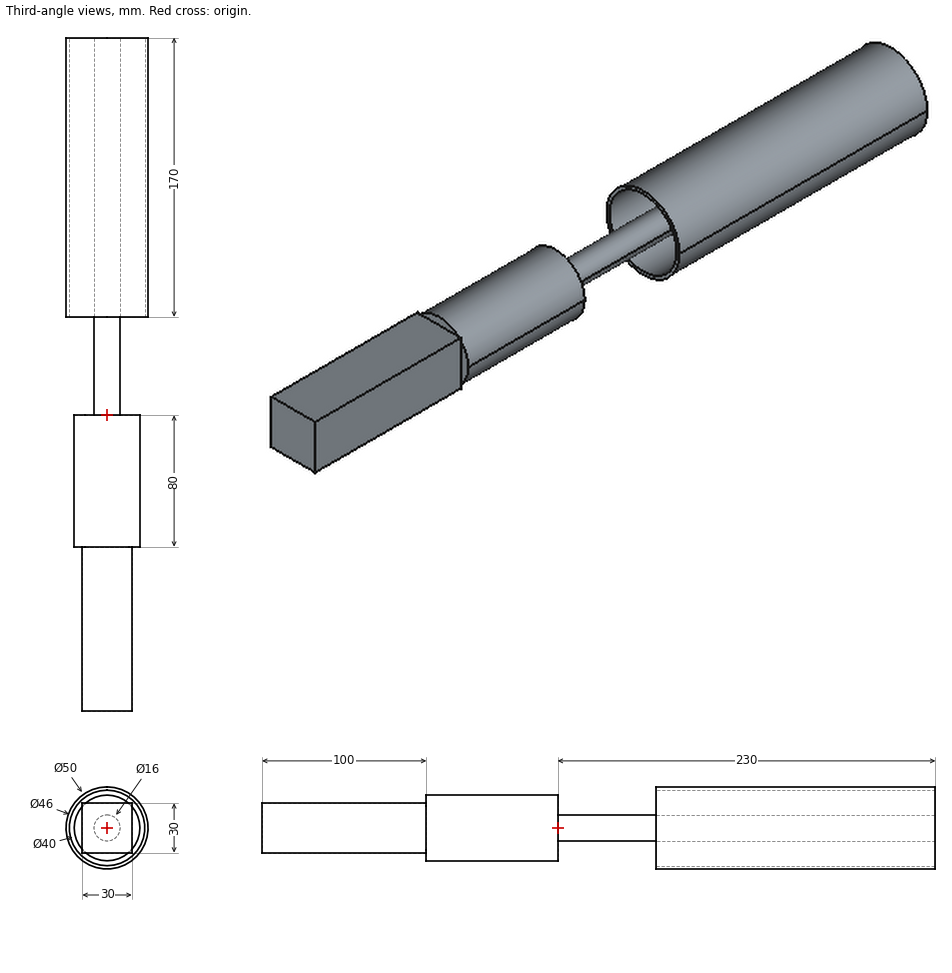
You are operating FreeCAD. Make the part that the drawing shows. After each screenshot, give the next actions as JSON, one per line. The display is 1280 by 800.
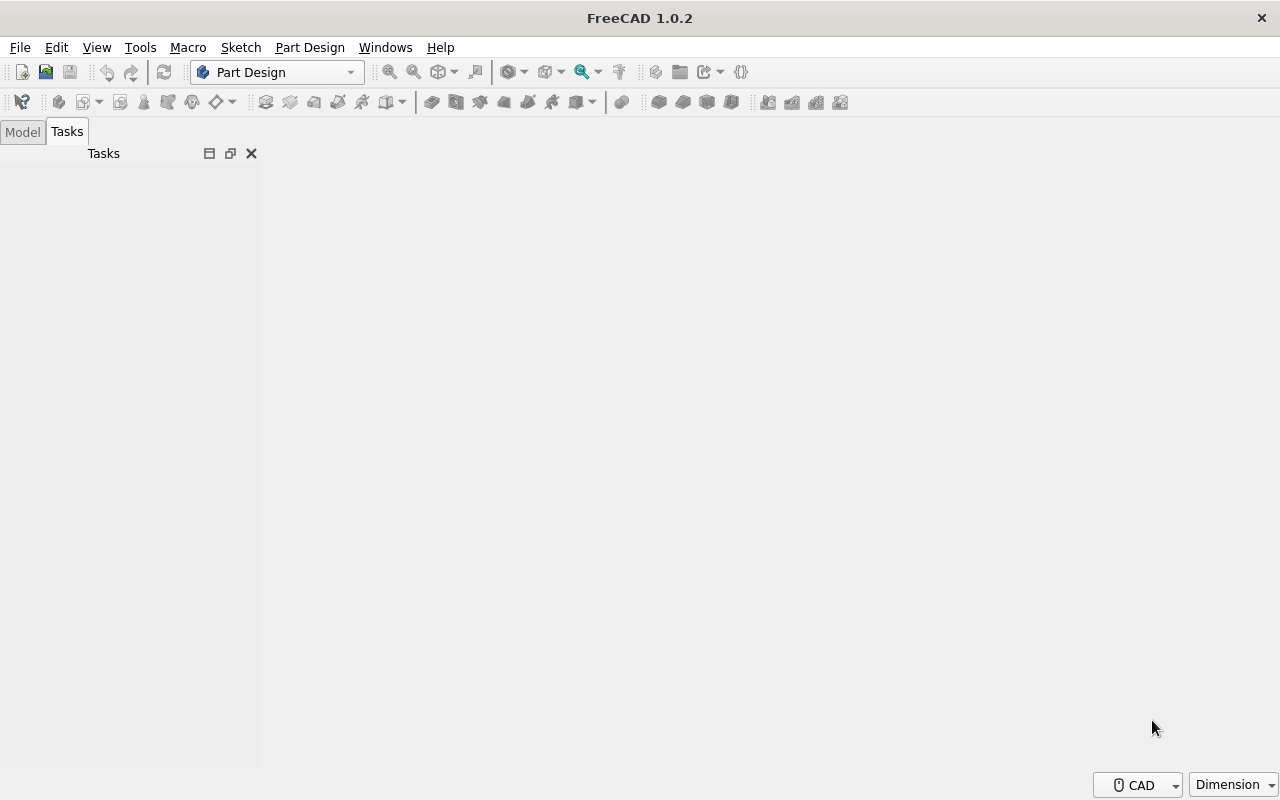
{"action": "left_click", "coordinate": [288, 72]}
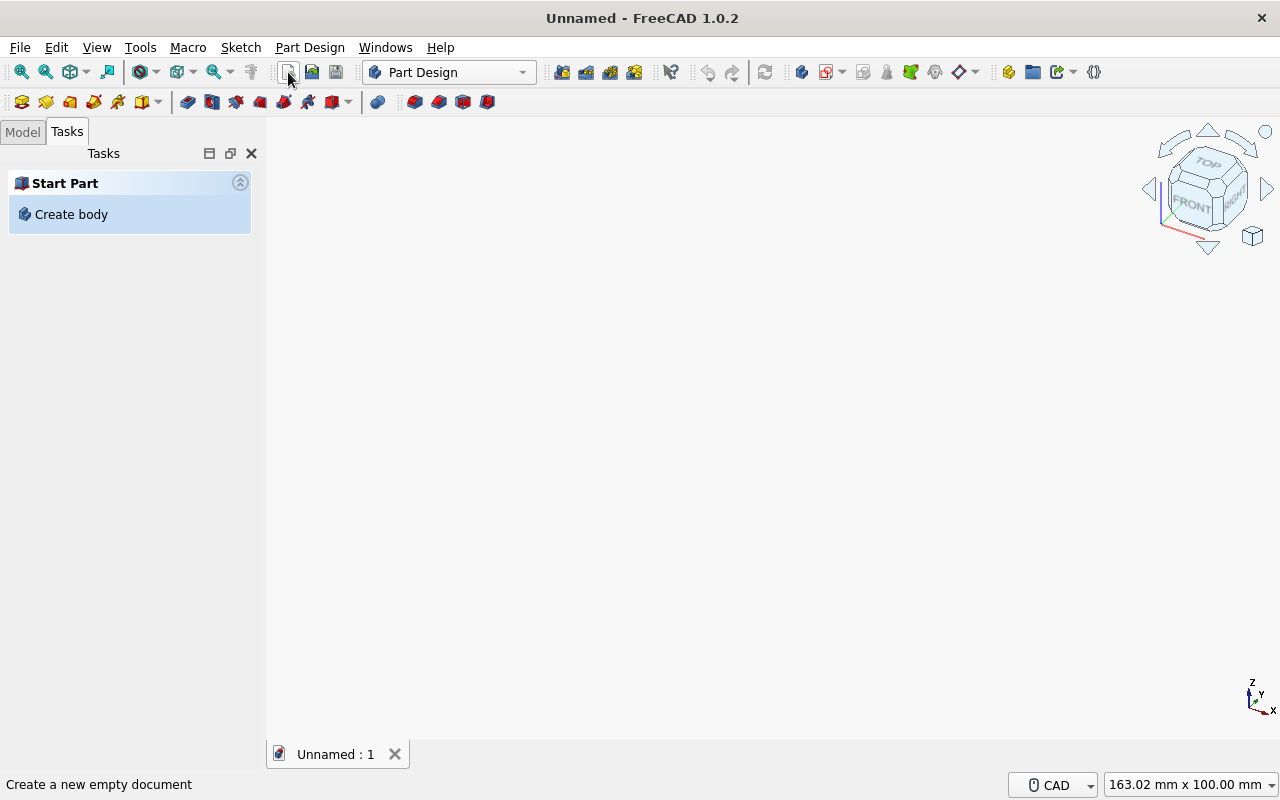
{"action": "left_click", "coordinate": [826, 72]}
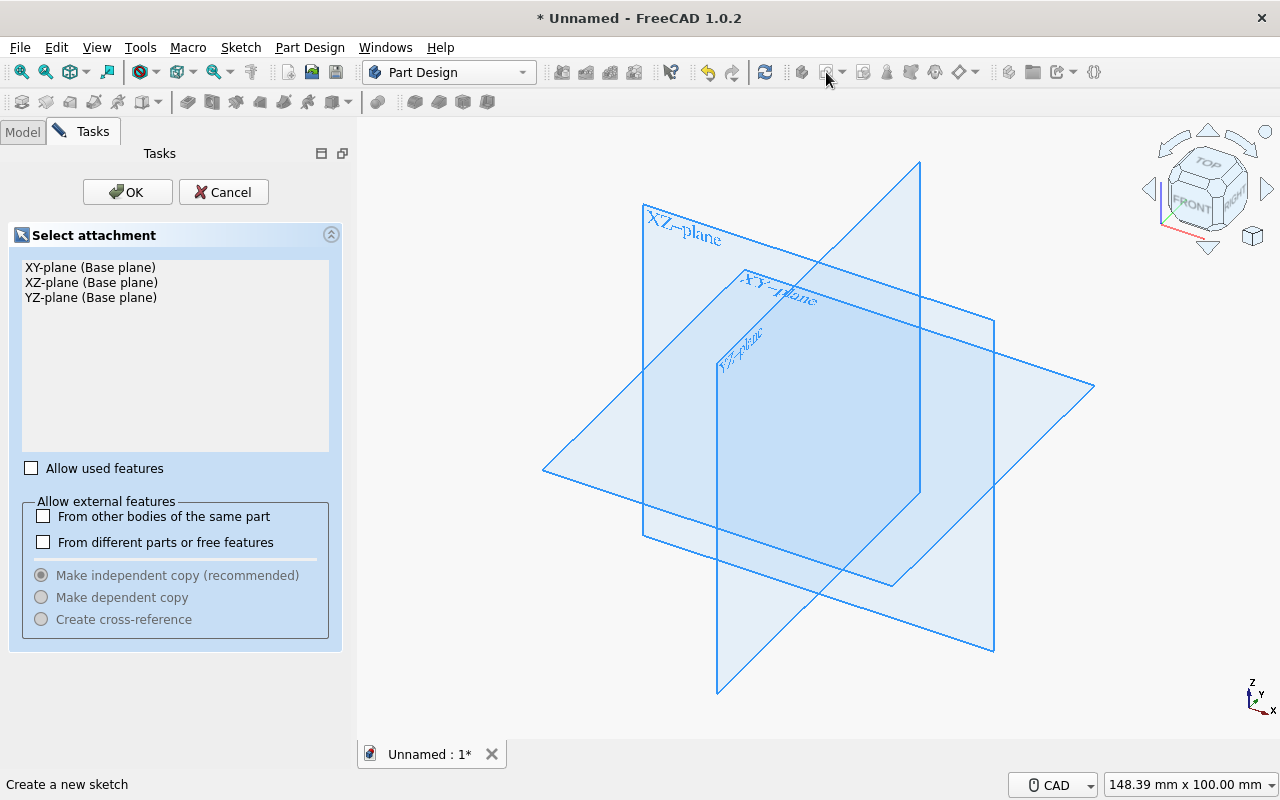
{"action": "left_click", "coordinate": [82, 282]}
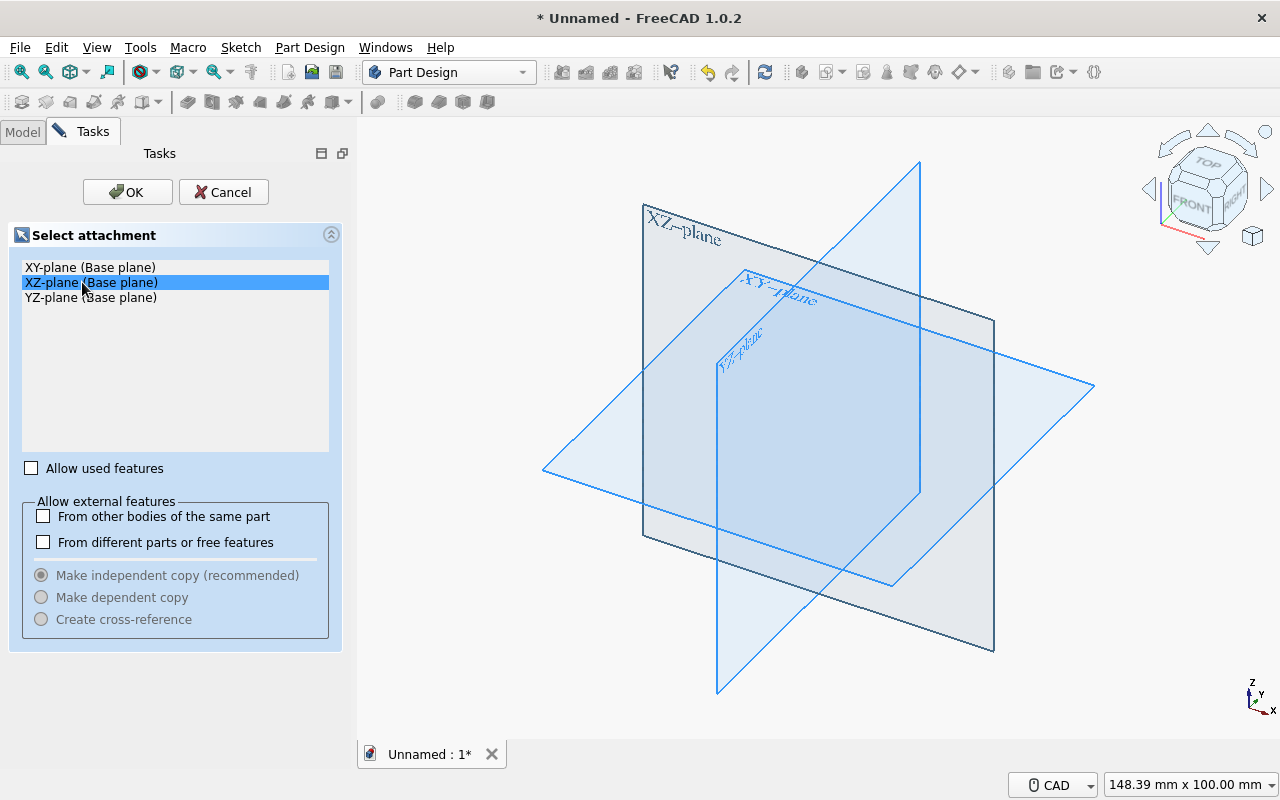
{"action": "left_click", "coordinate": [128, 192]}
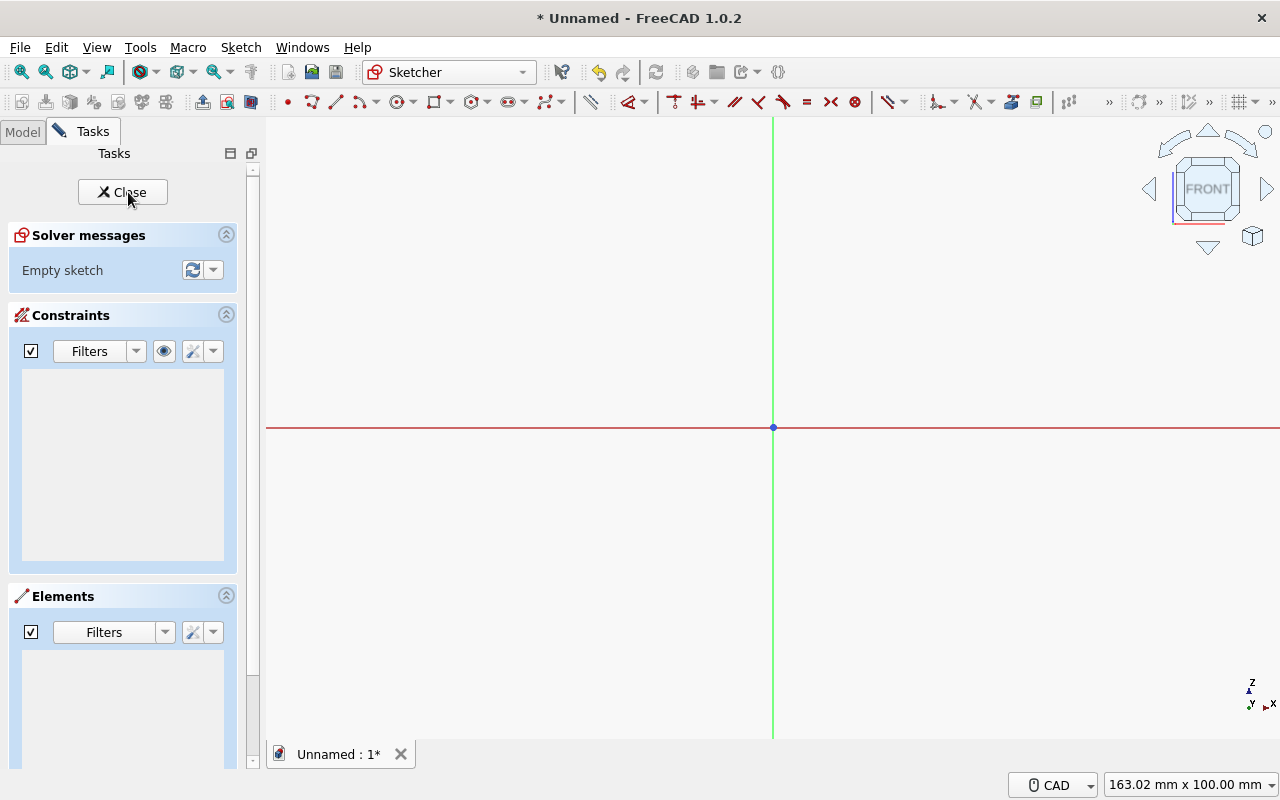
{"action": "scroll", "coordinate": [795, 428], "scroll_direction": "up", "scroll_amount": 7}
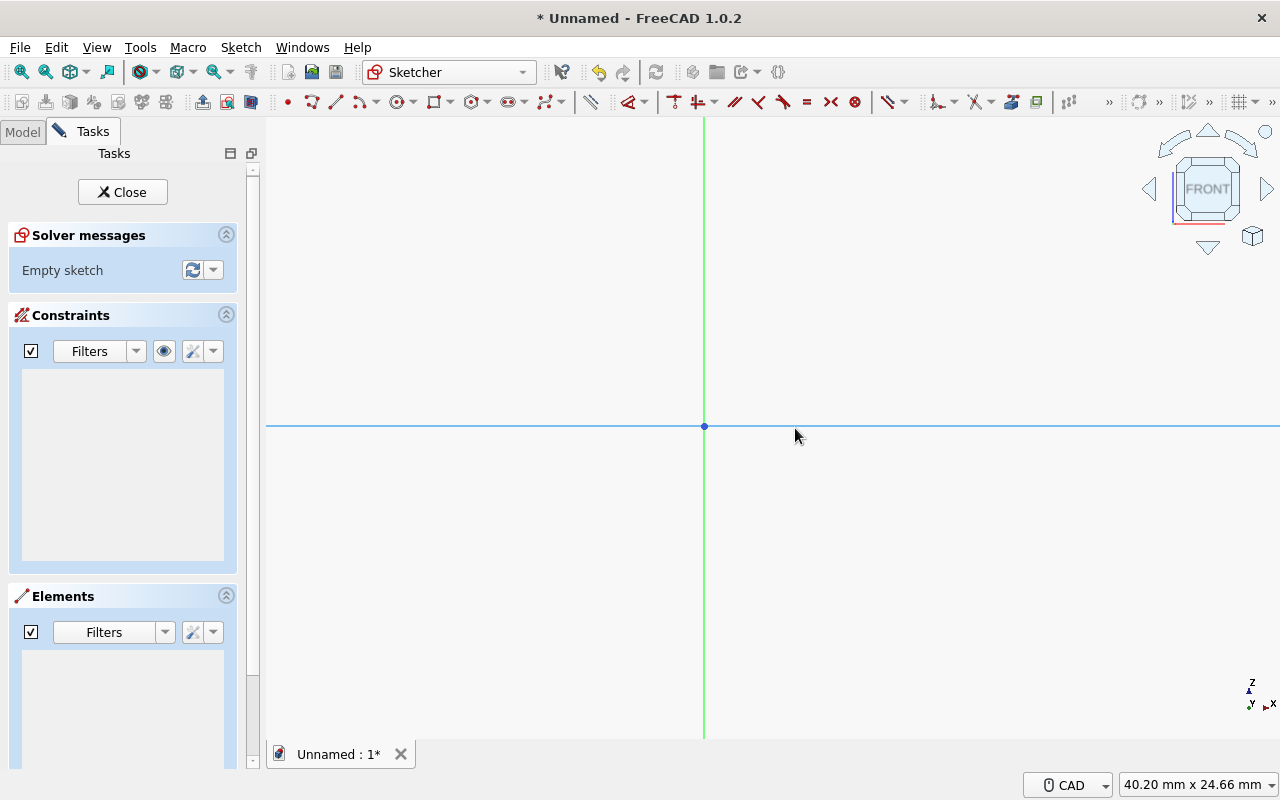
{"action": "left_click", "coordinate": [398, 102]}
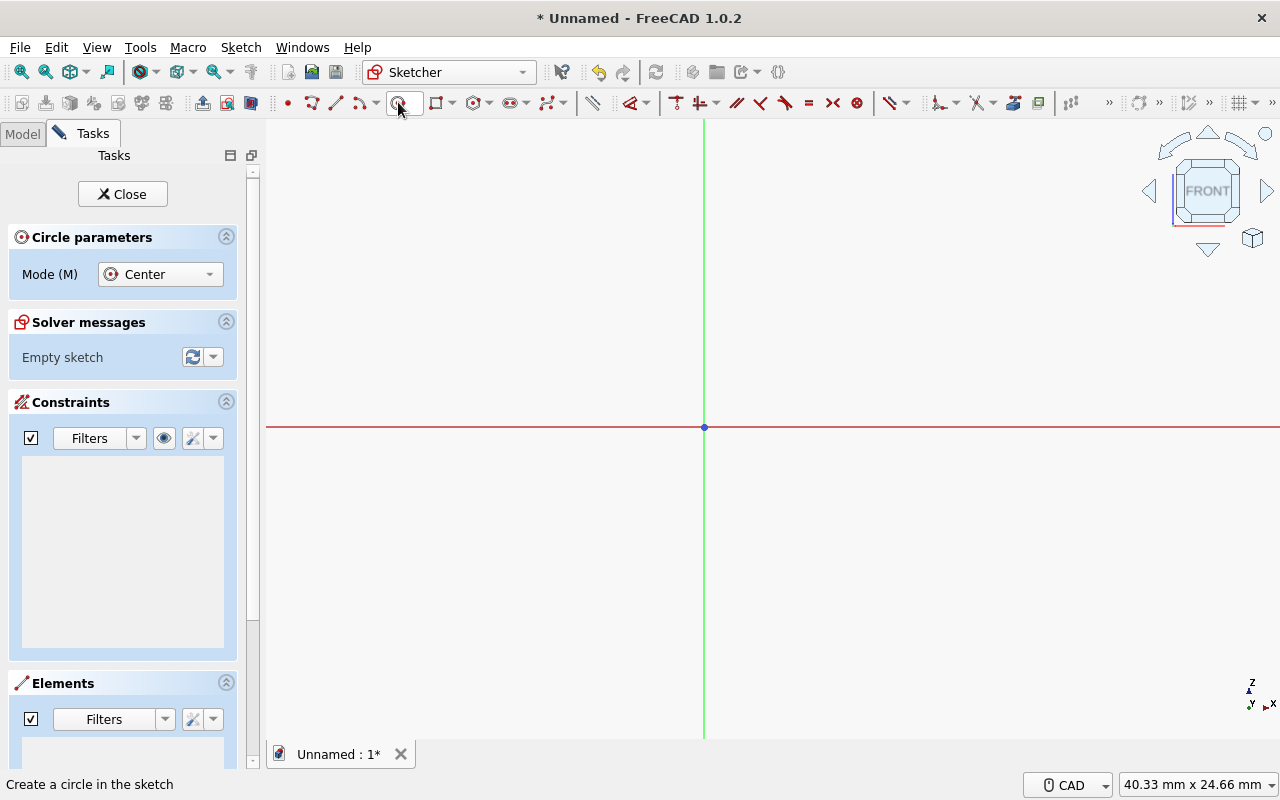
{"action": "left_click", "coordinate": [704, 427]}
{"action": "mouse_move", "coordinate": [847, 285]}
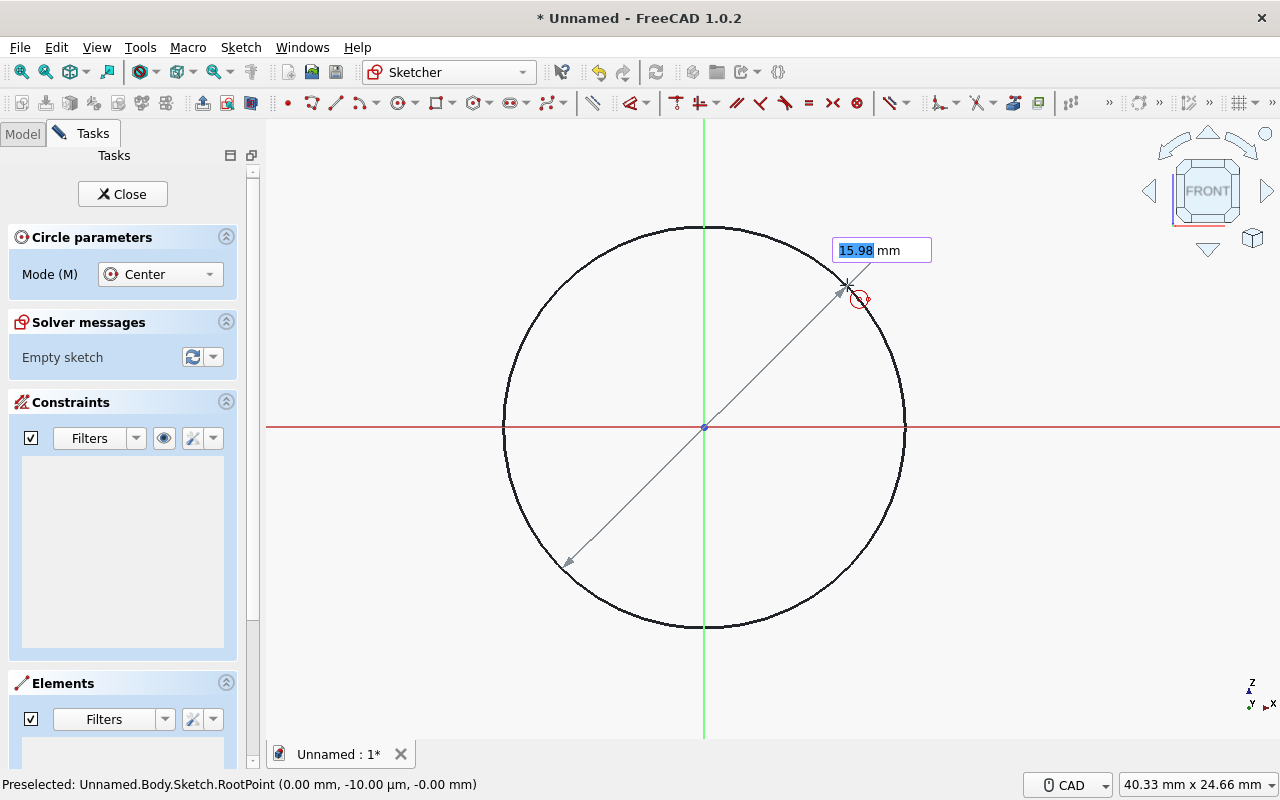
{"action": "type", "text": "16"}
{"action": "key", "text": "Return"}
{"action": "key", "text": "Escape"}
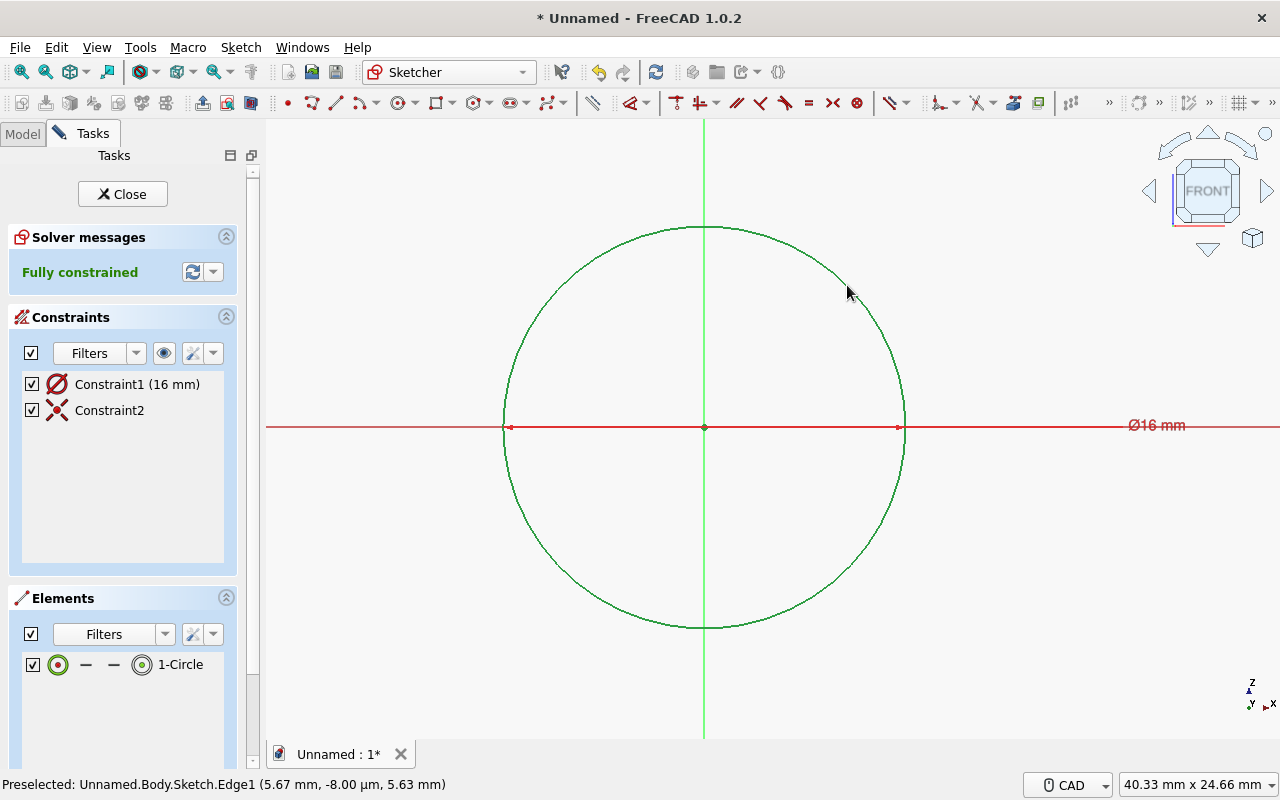
{"action": "left_click", "coordinate": [123, 194]}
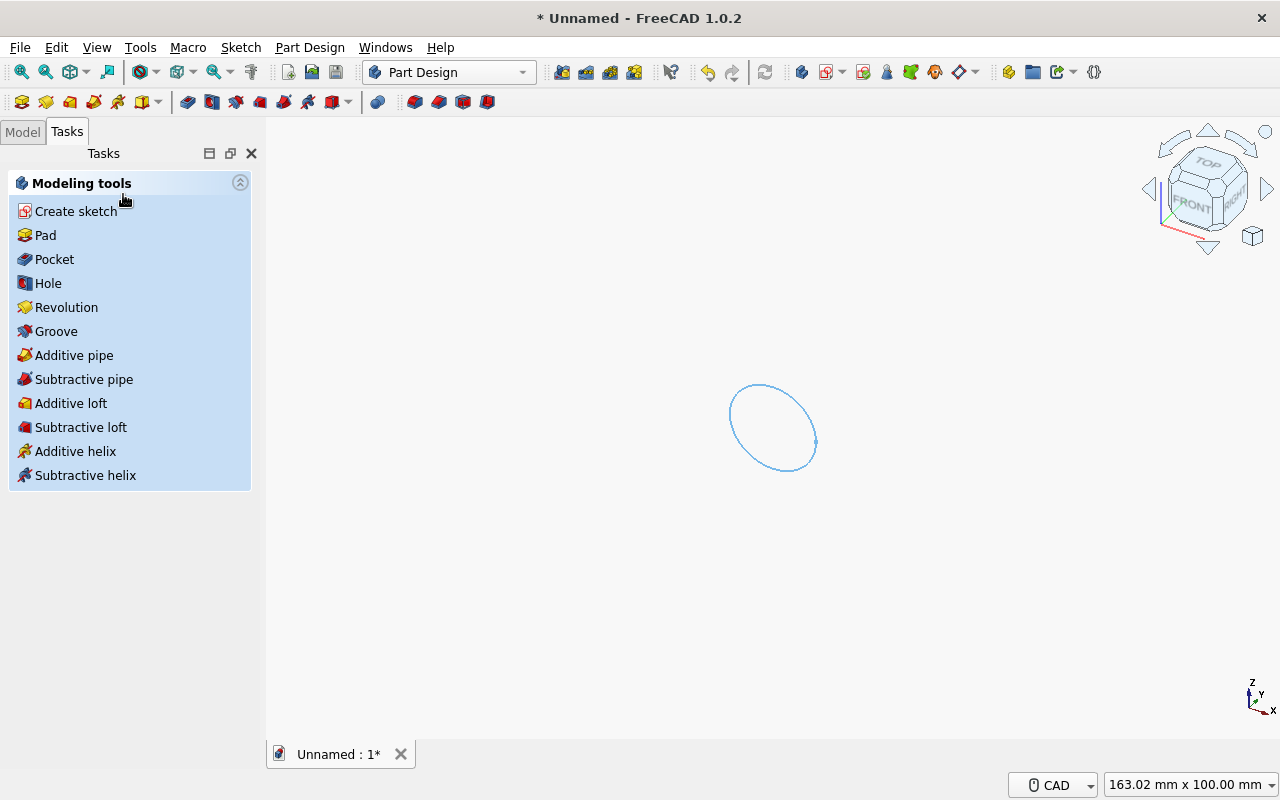
{"action": "left_click", "coordinate": [22, 102]}